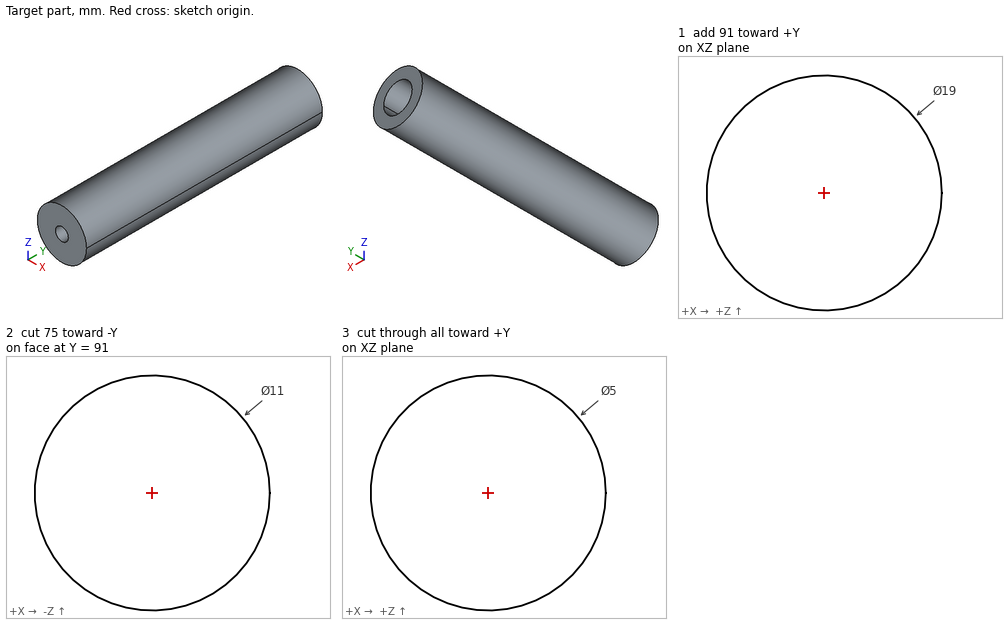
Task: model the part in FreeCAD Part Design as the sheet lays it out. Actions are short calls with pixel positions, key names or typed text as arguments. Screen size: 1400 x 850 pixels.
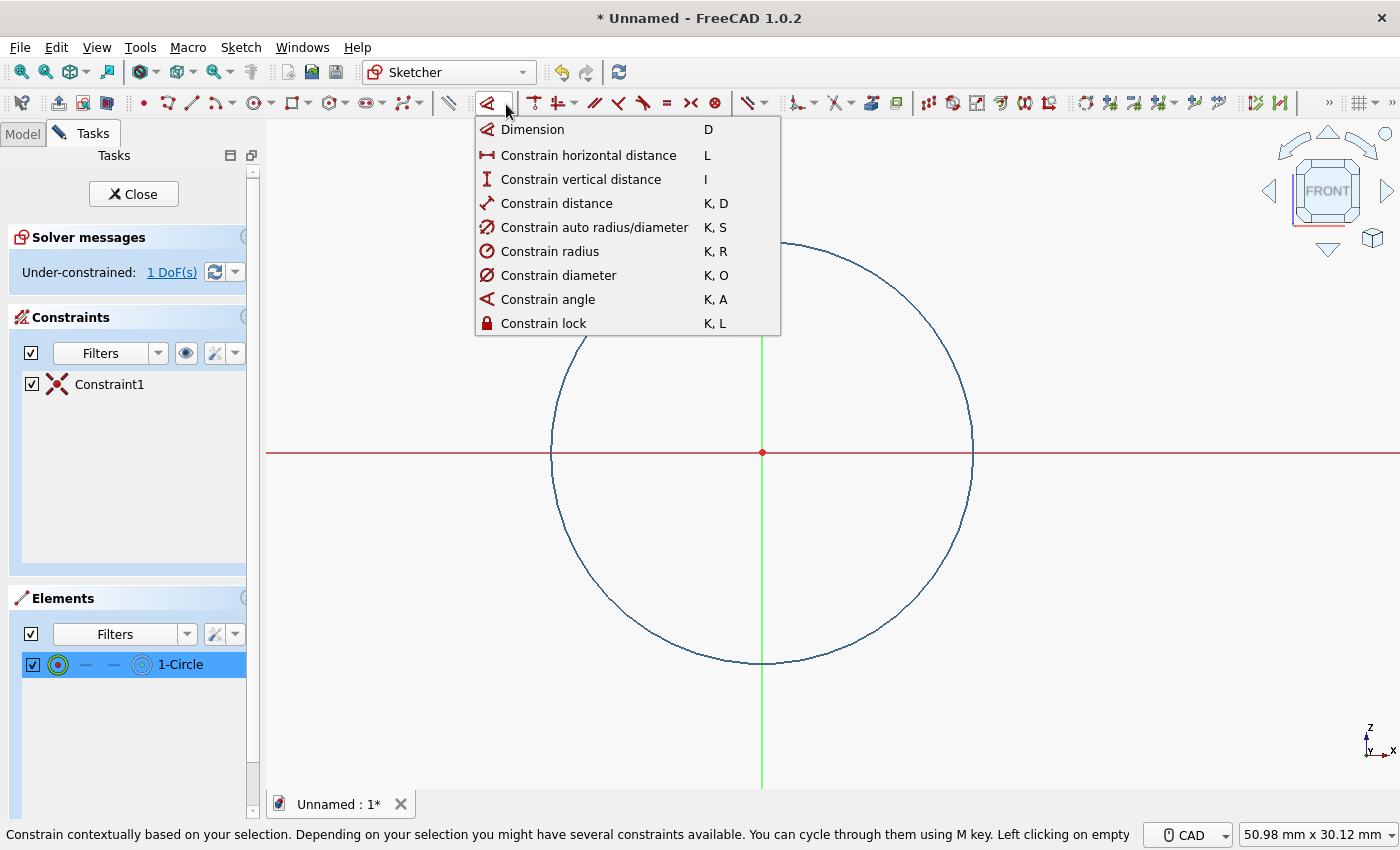
click(628, 275)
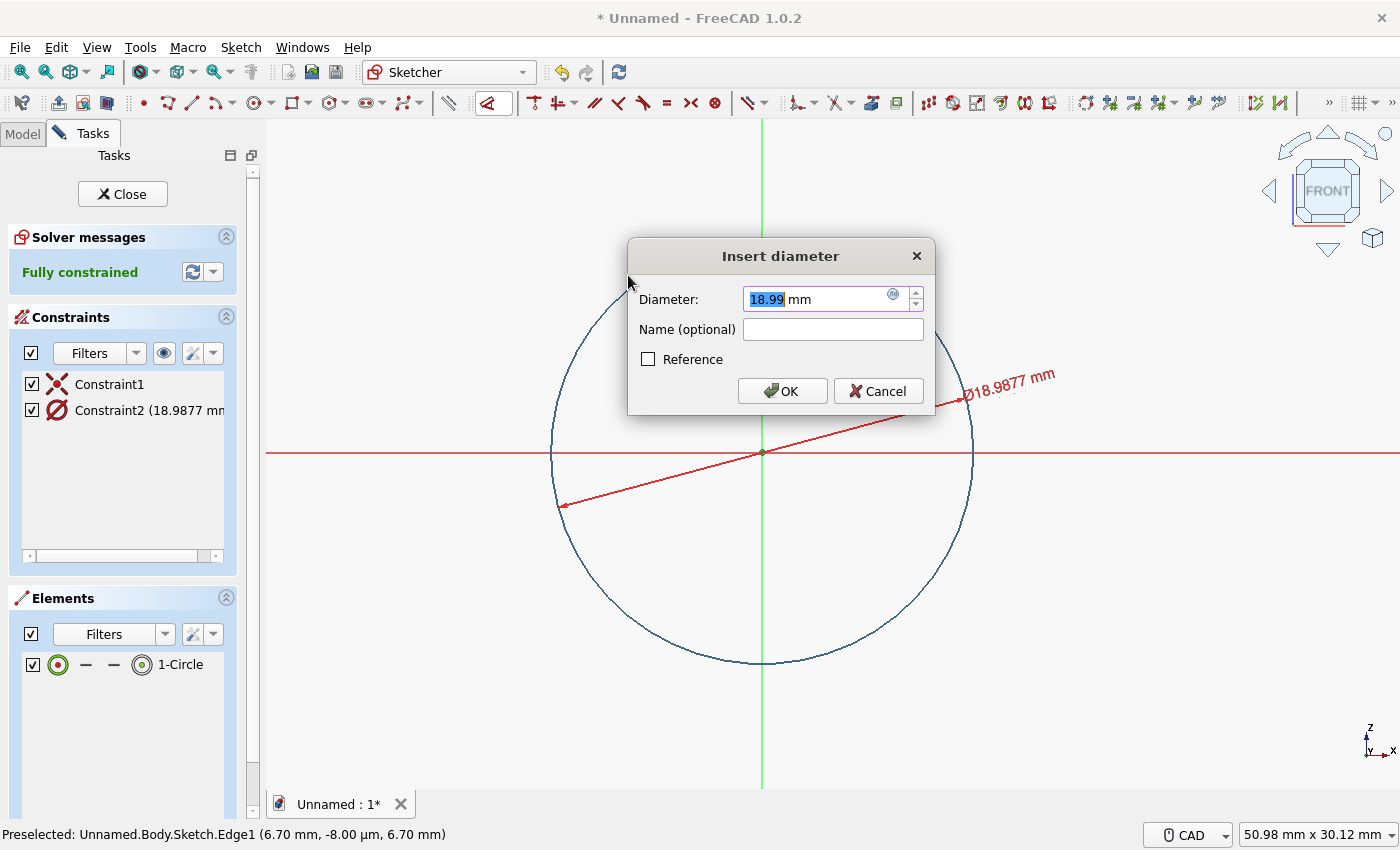
text(19)
key(Return)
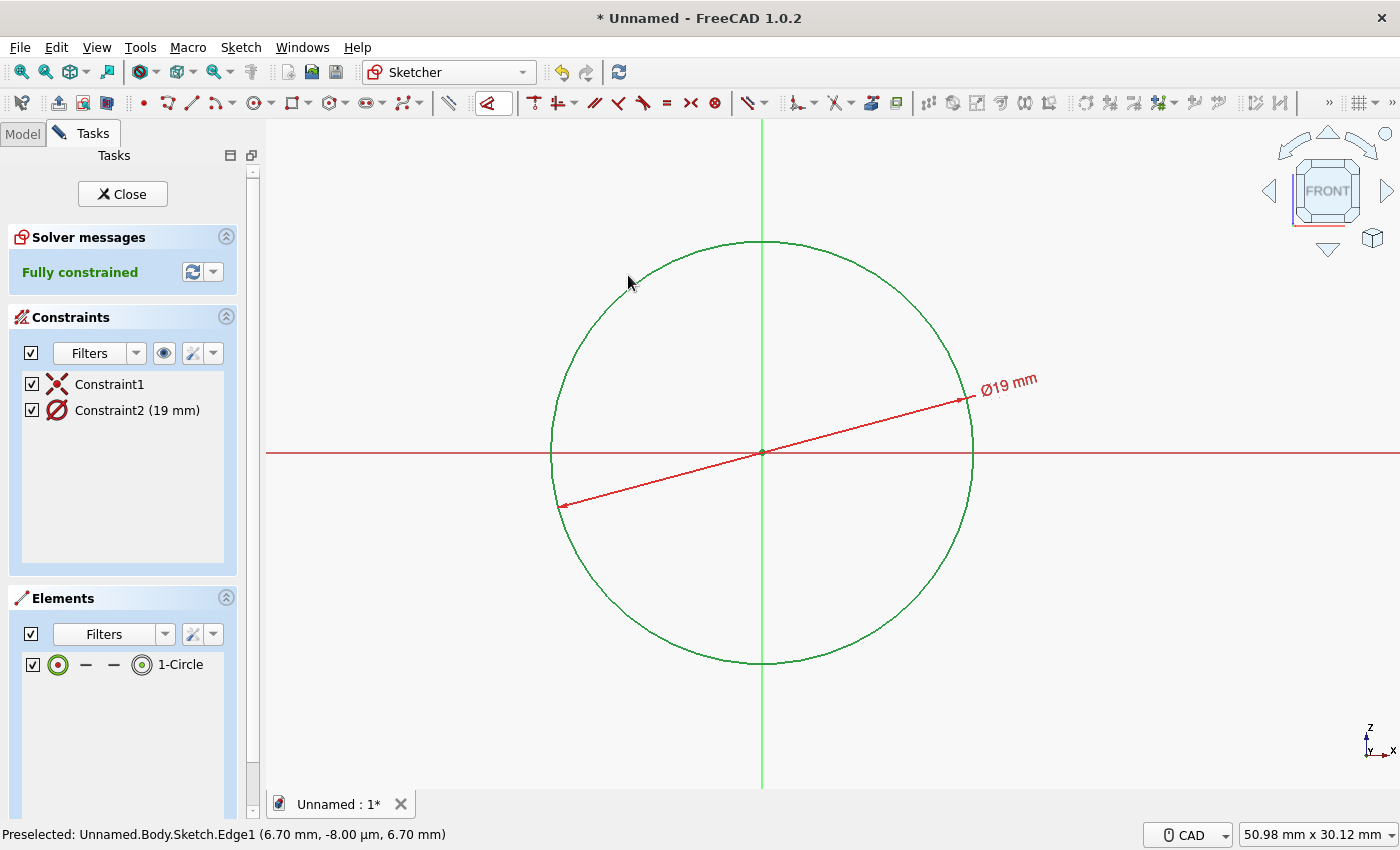
click(123, 194)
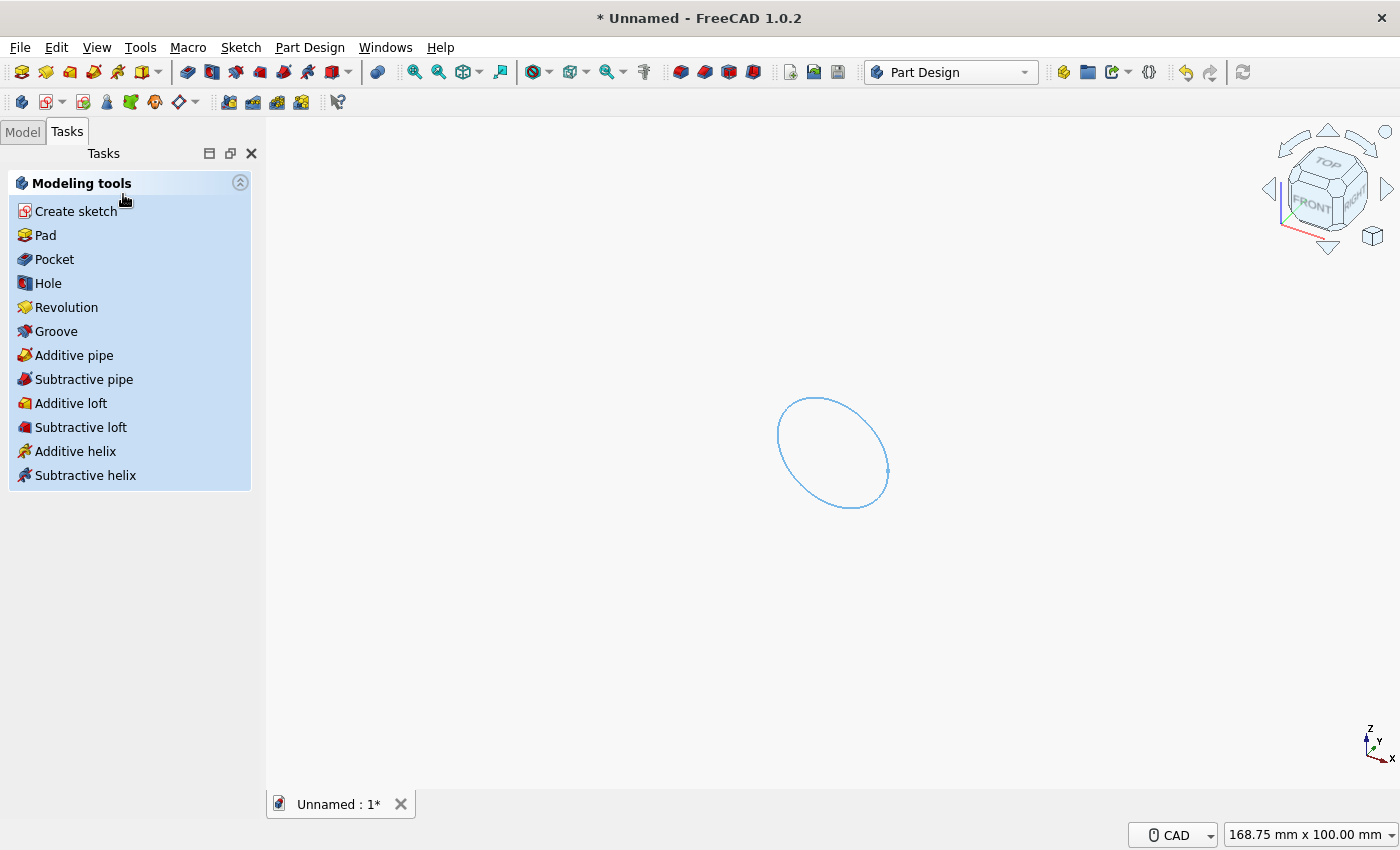
click(22, 72)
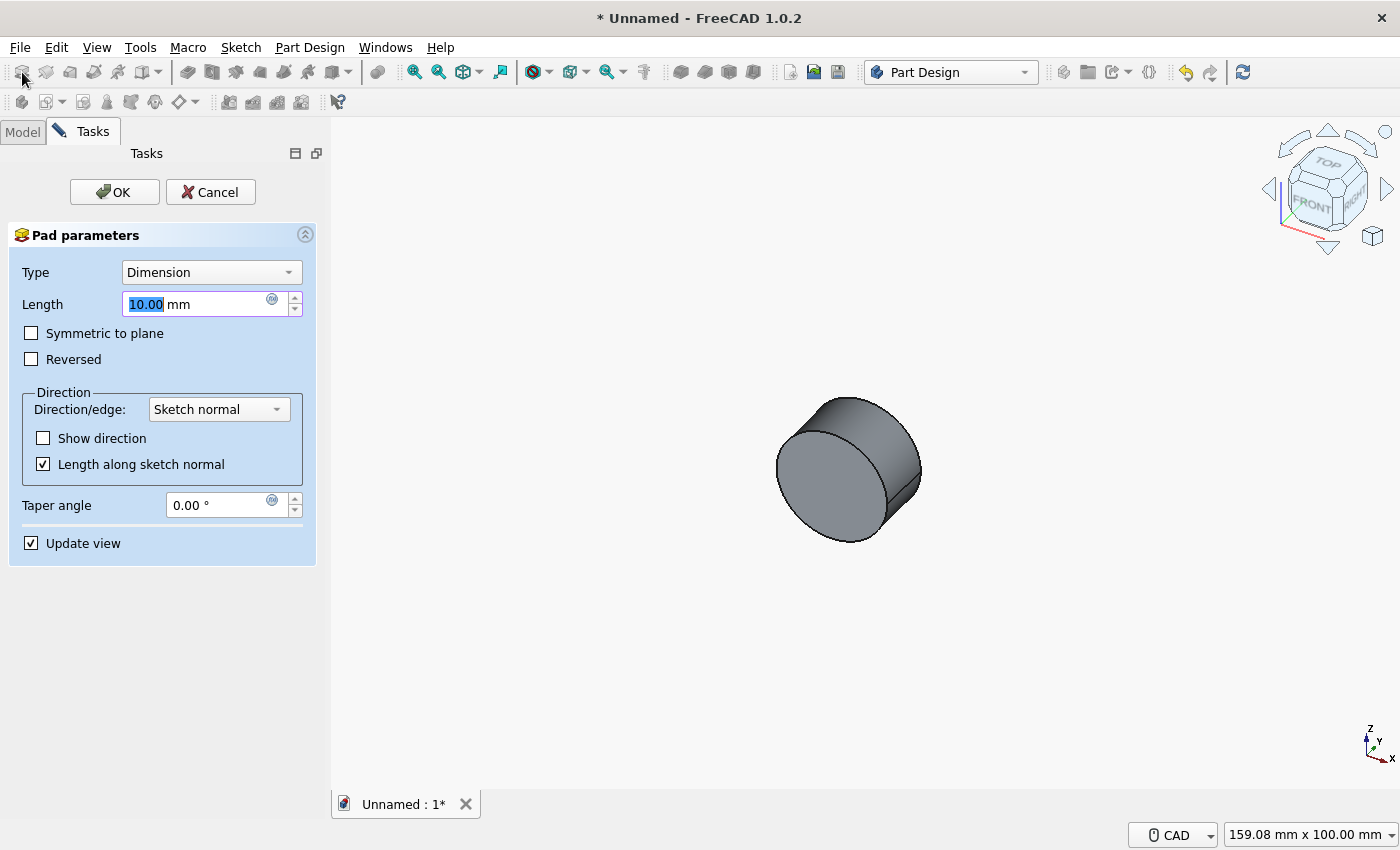
text(91)
key(Tab)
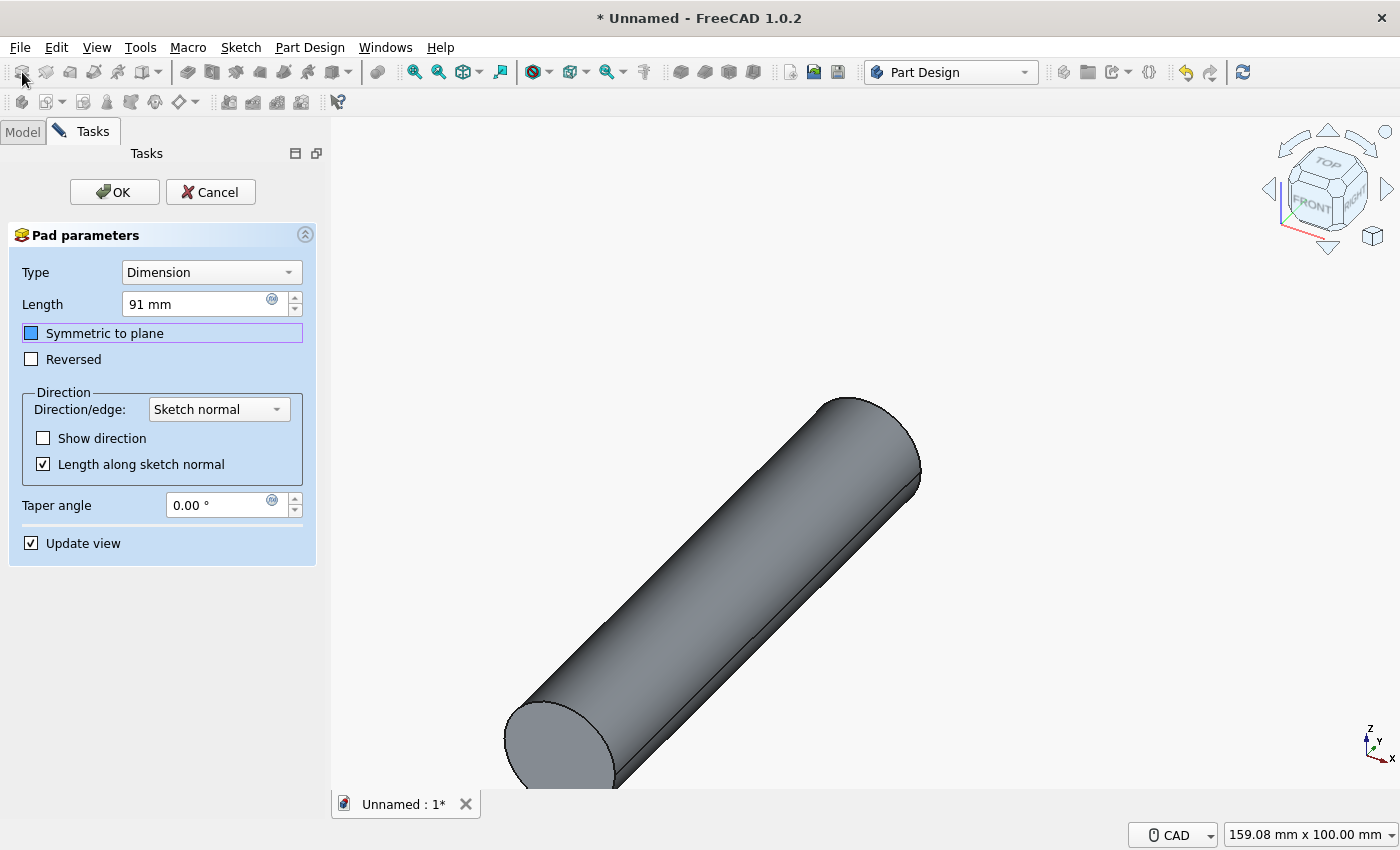
click(30, 359)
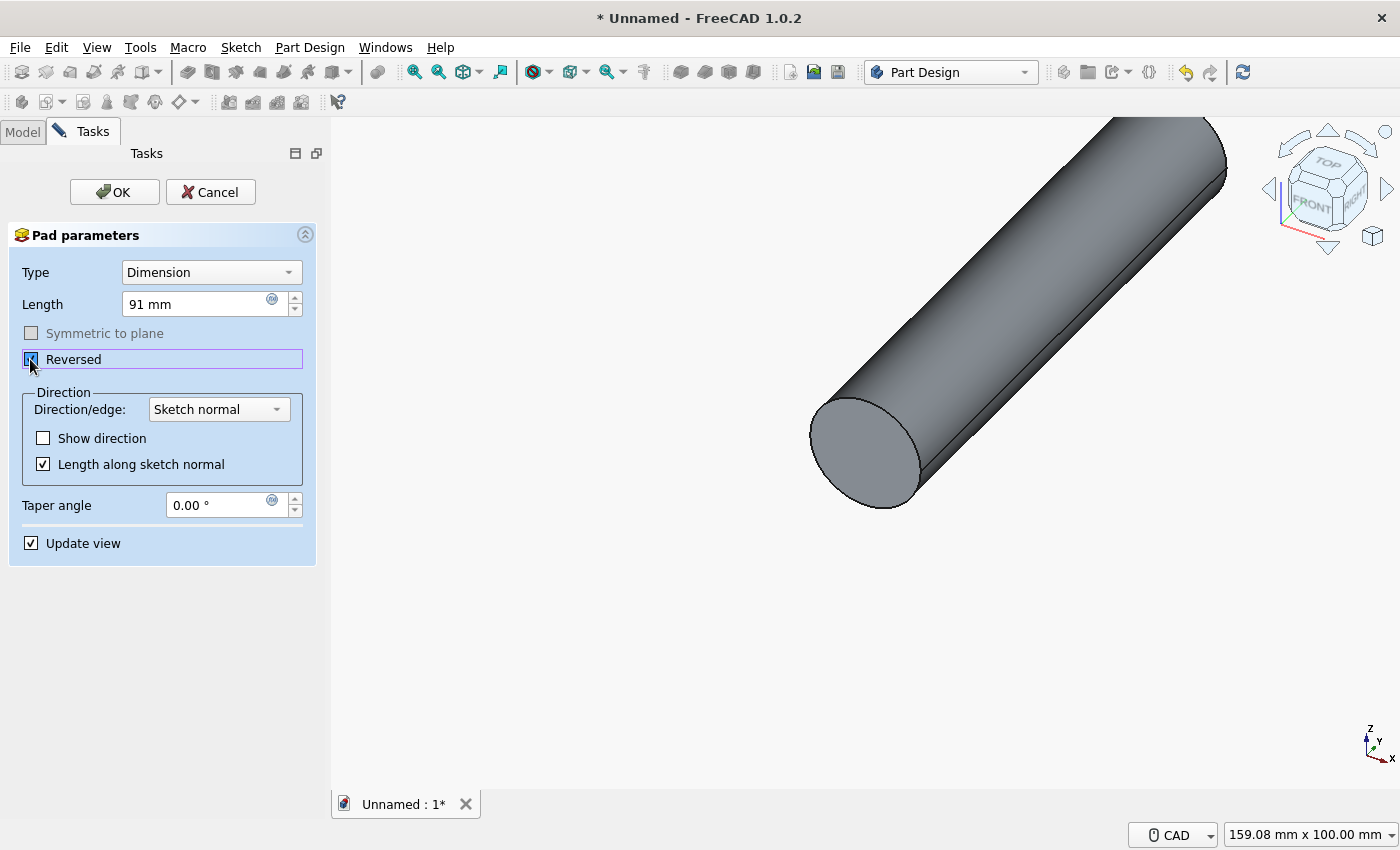
click(115, 192)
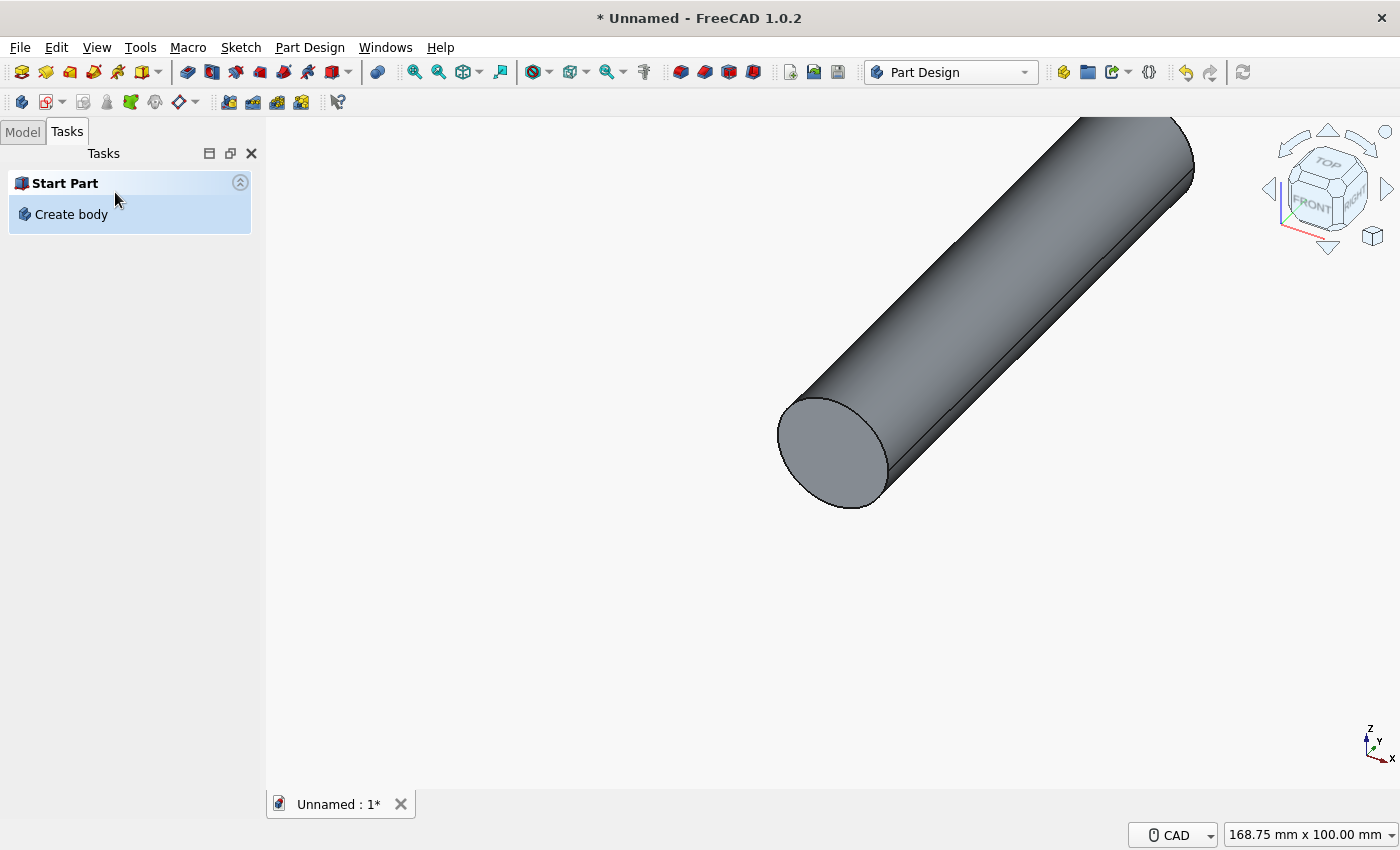
key(v)
key(f)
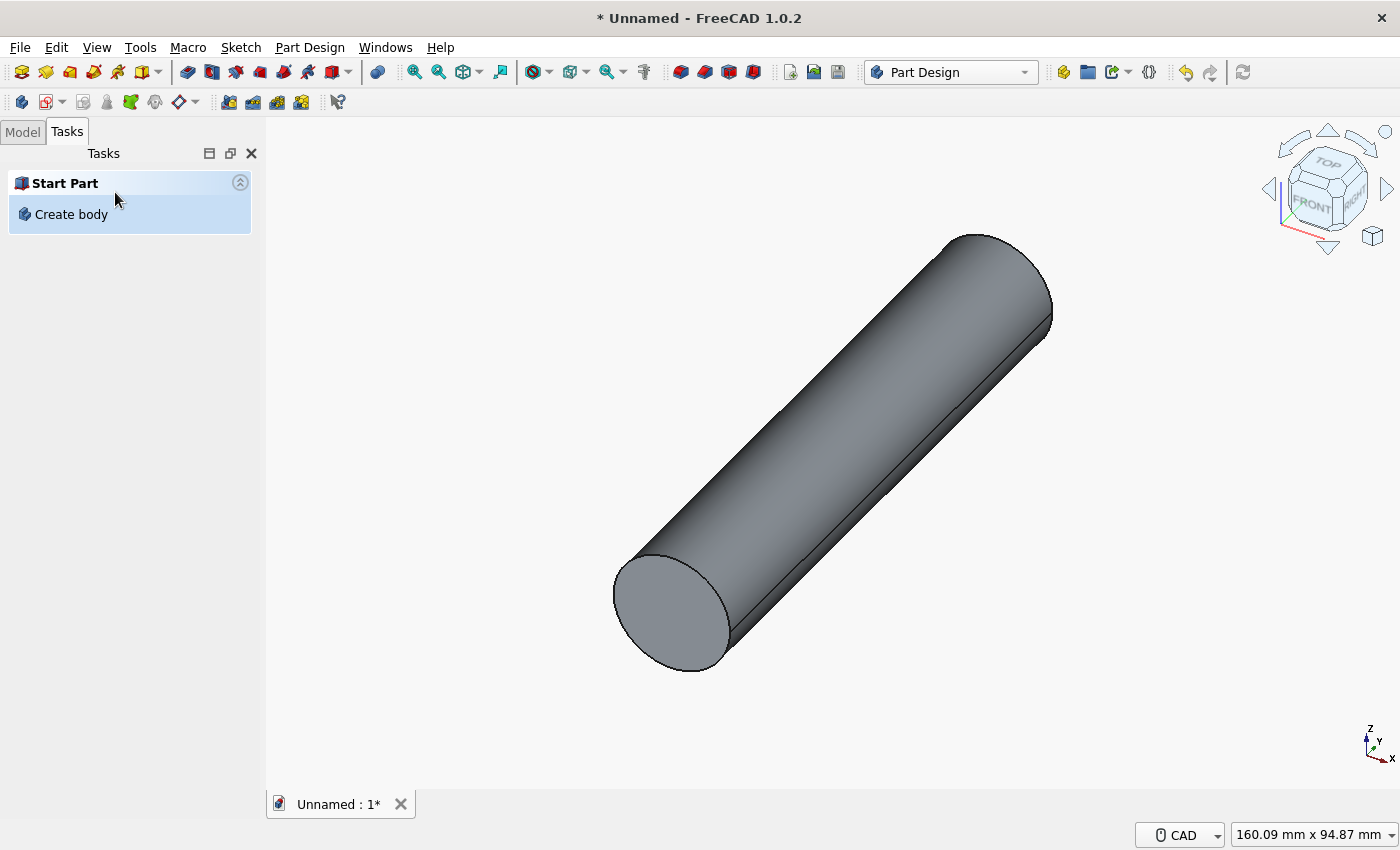
key(4)